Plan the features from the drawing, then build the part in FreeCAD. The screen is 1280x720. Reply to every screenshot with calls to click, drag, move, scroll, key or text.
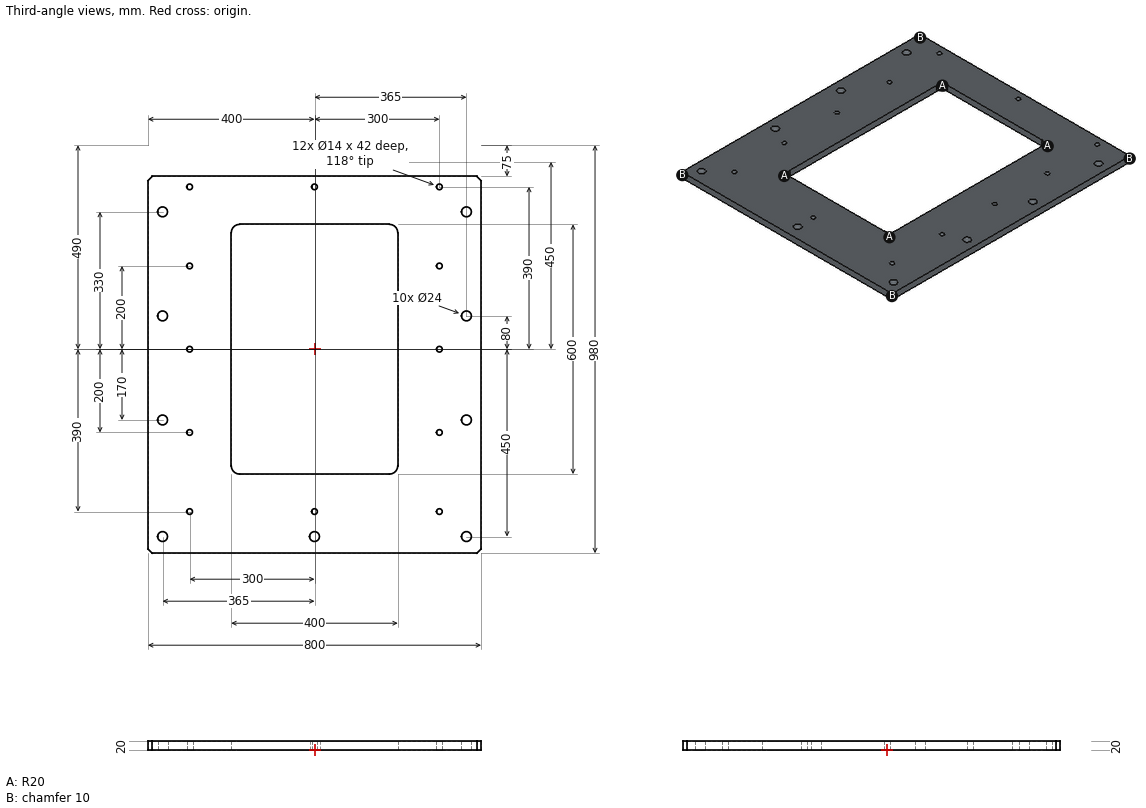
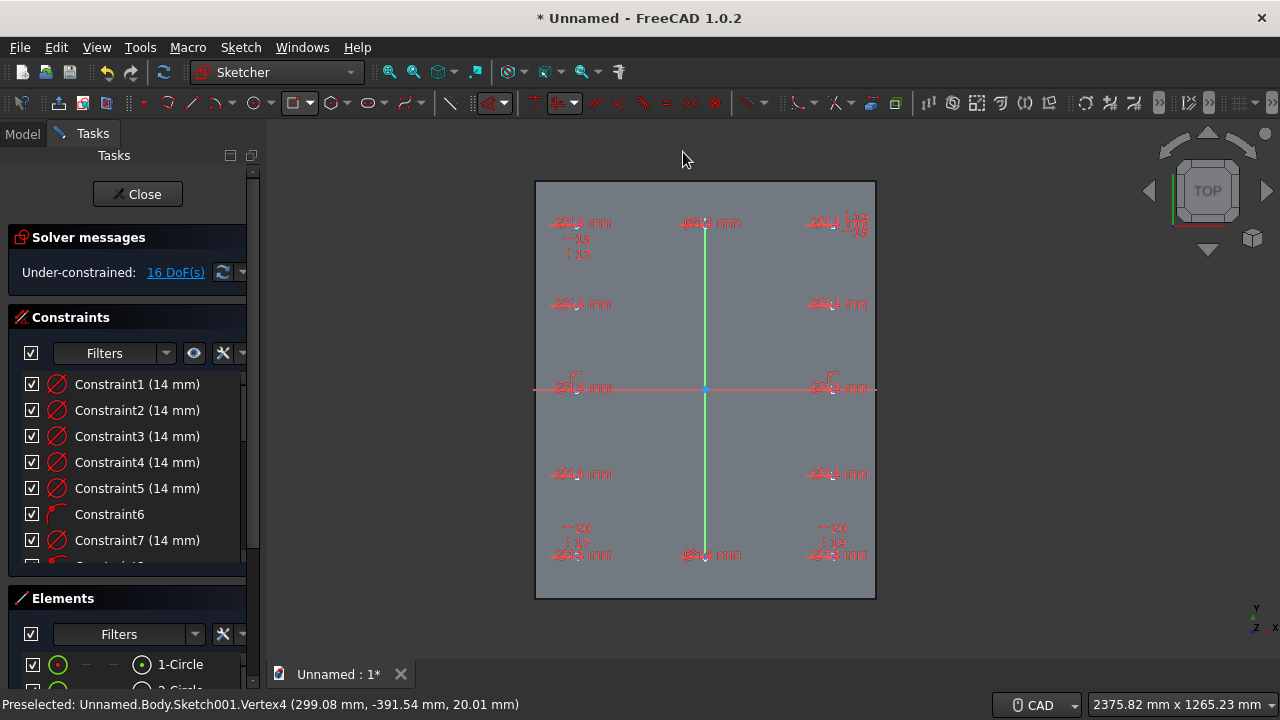
click(577, 557)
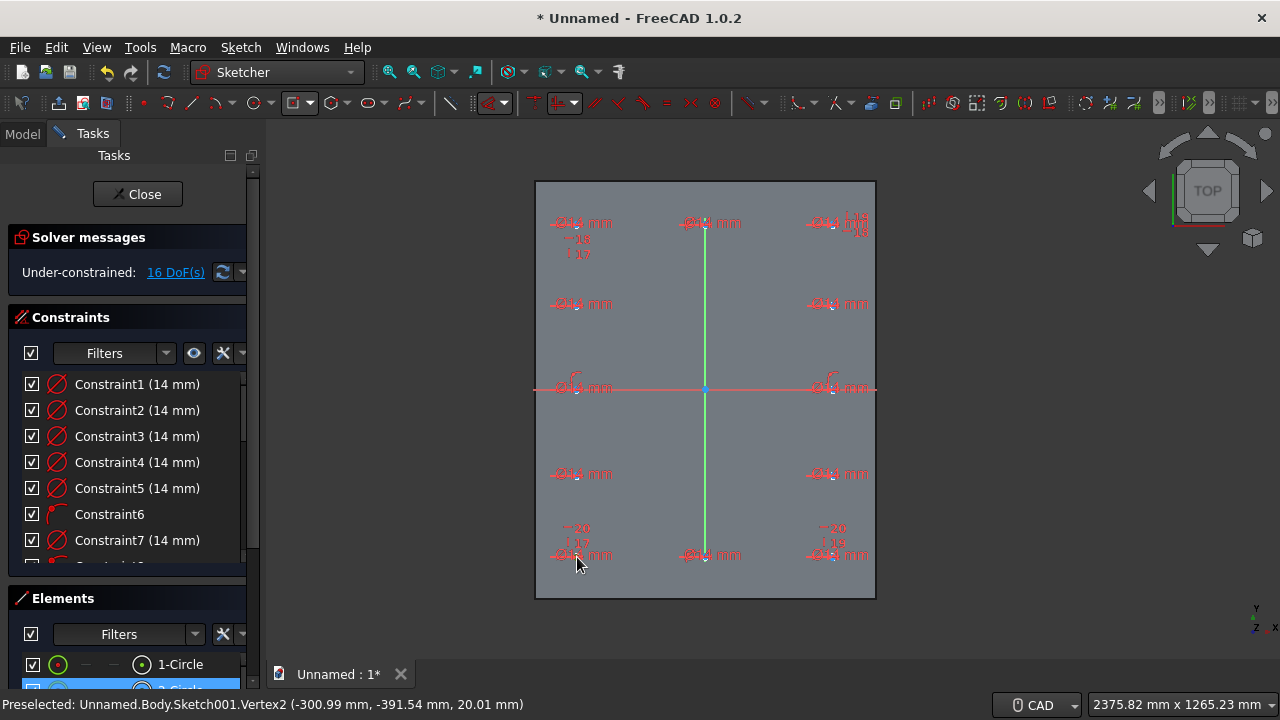
click(577, 390)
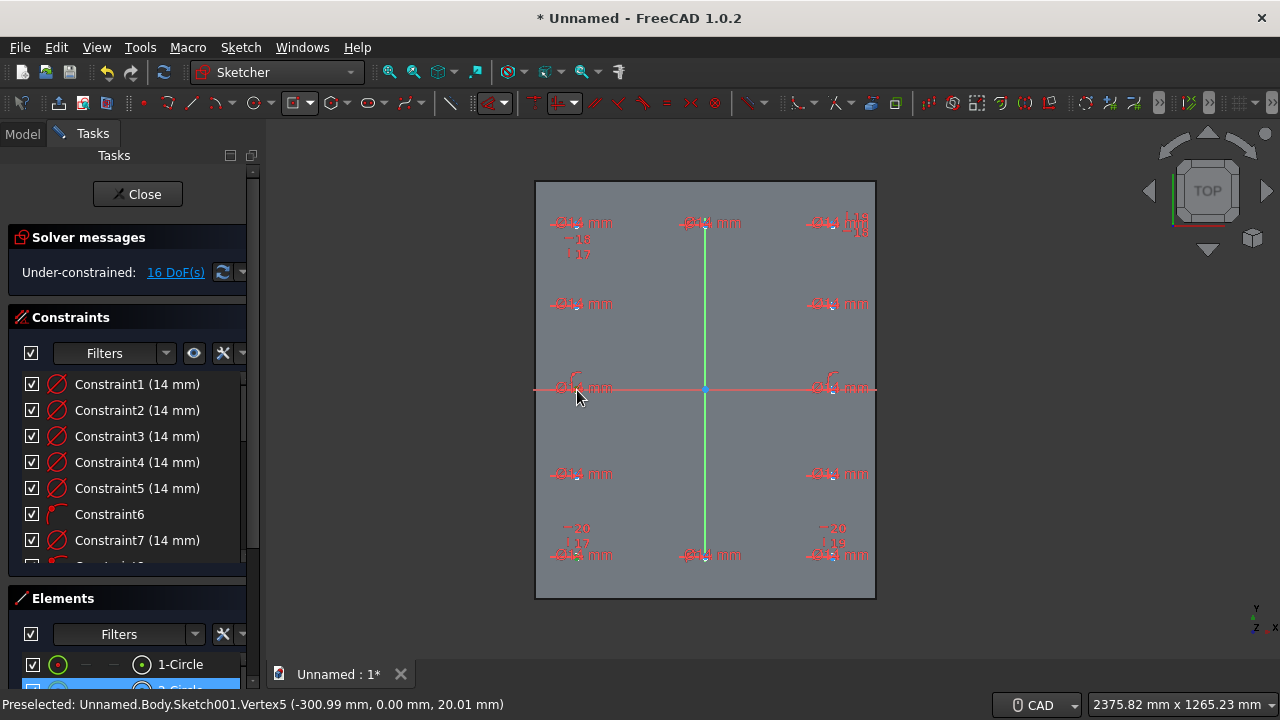
click(576, 104)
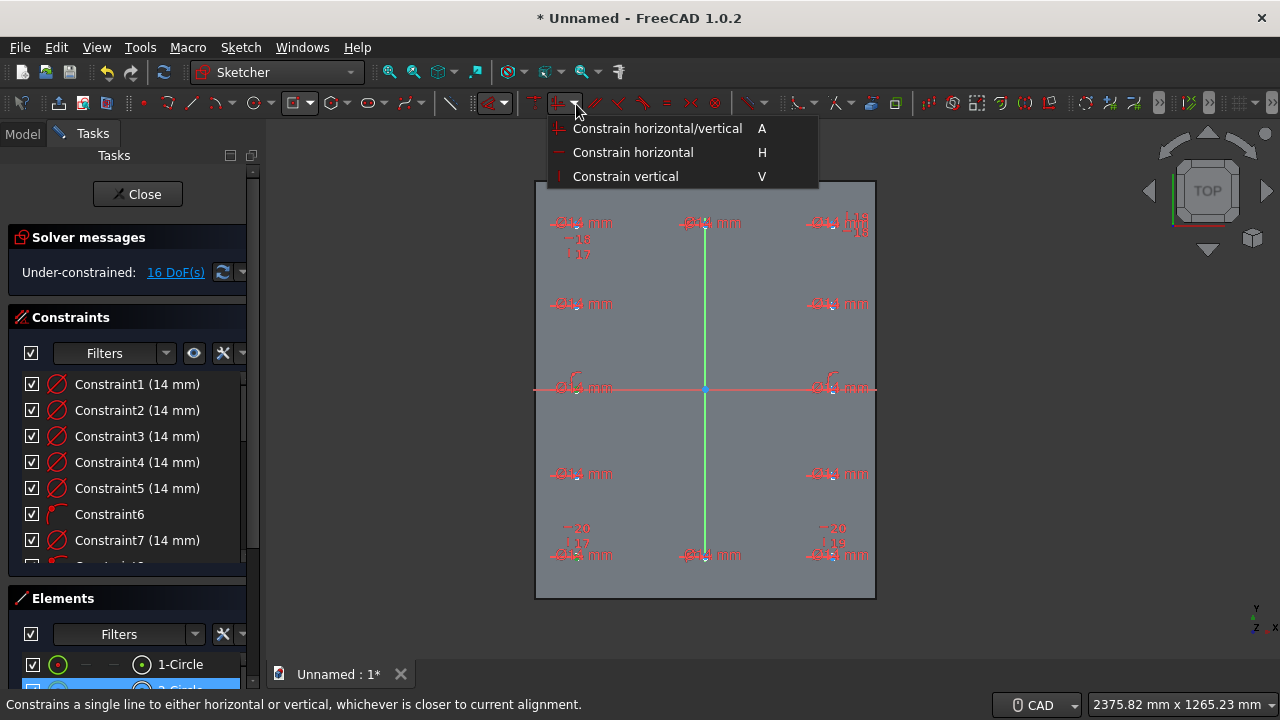
click(683, 176)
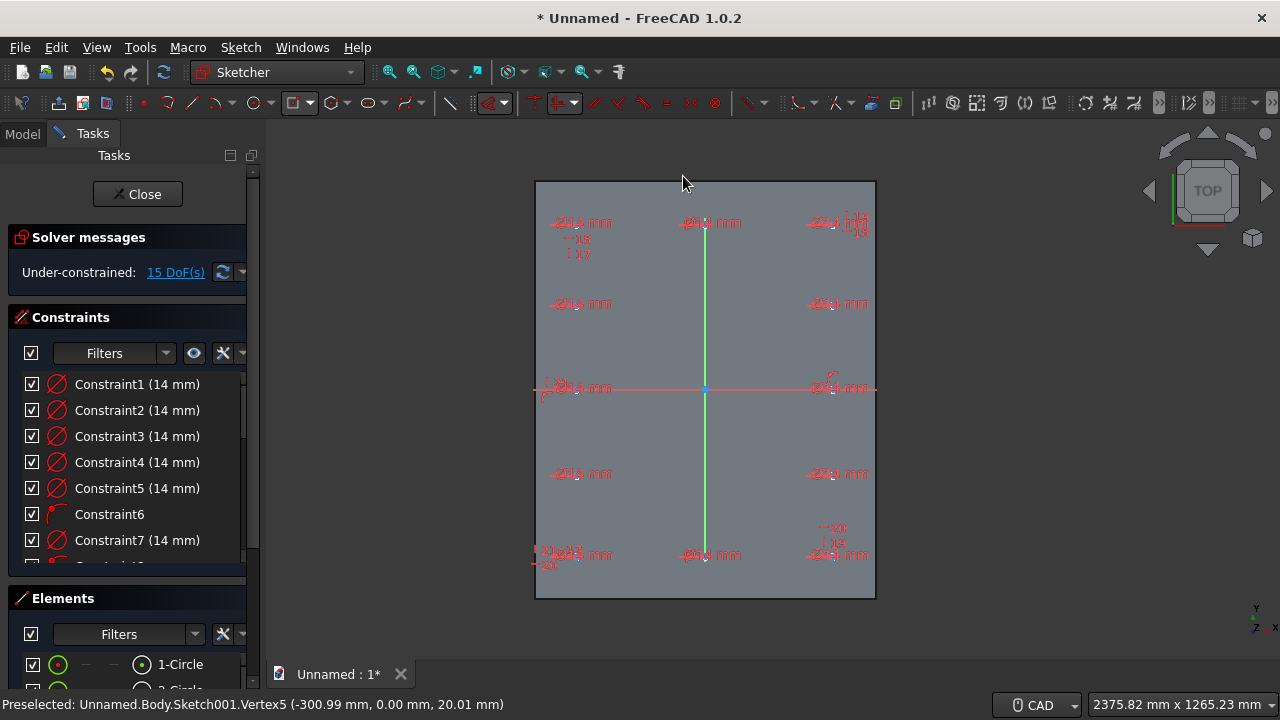
click(577, 557)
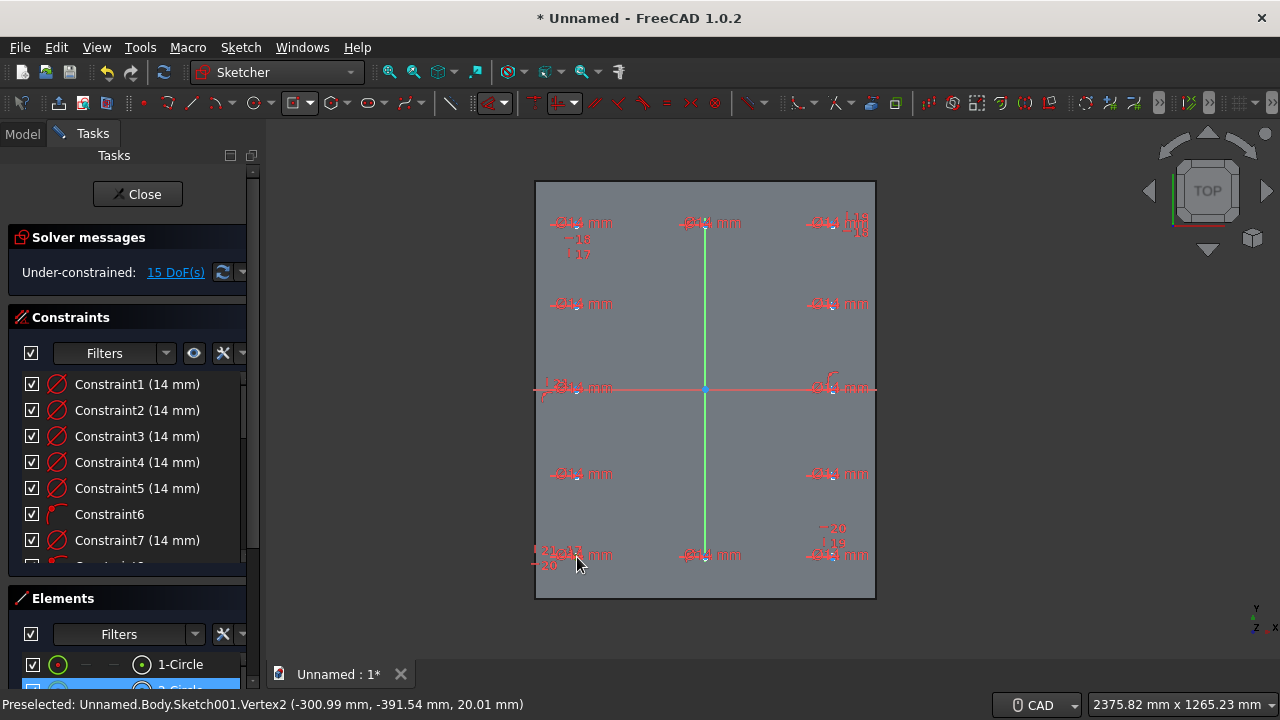
click(705, 557)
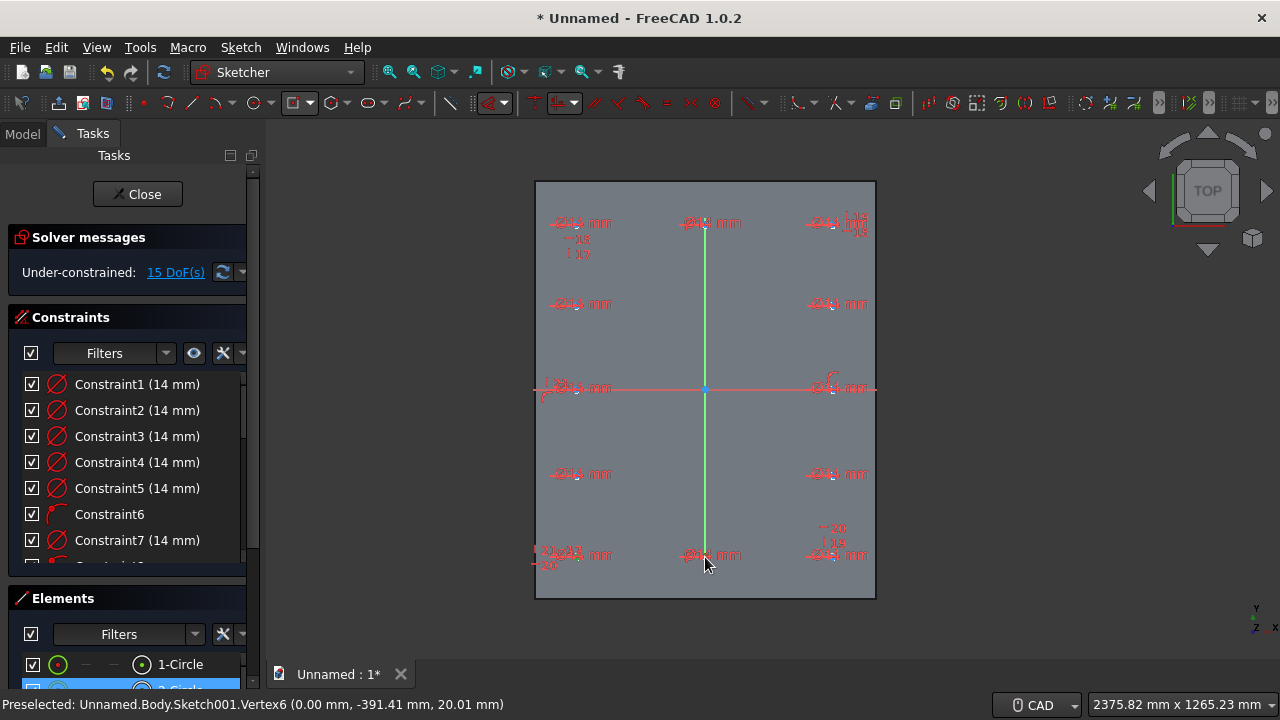
click(576, 104)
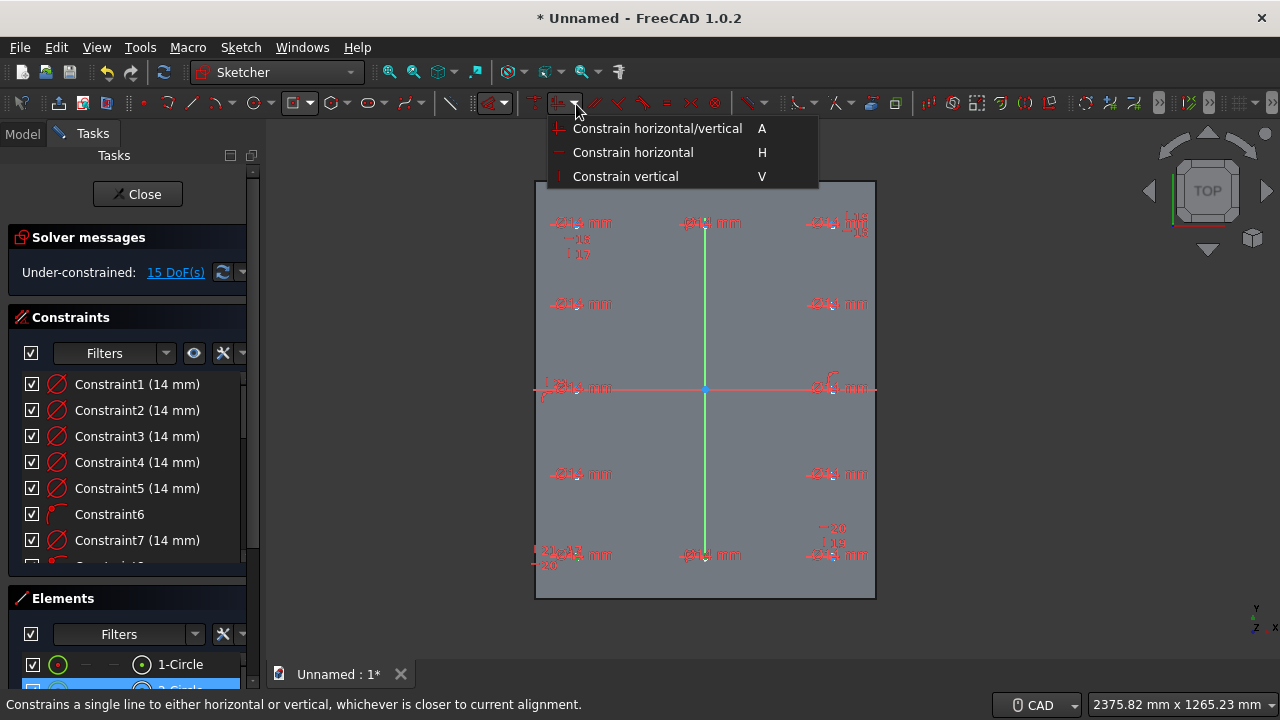
click(683, 152)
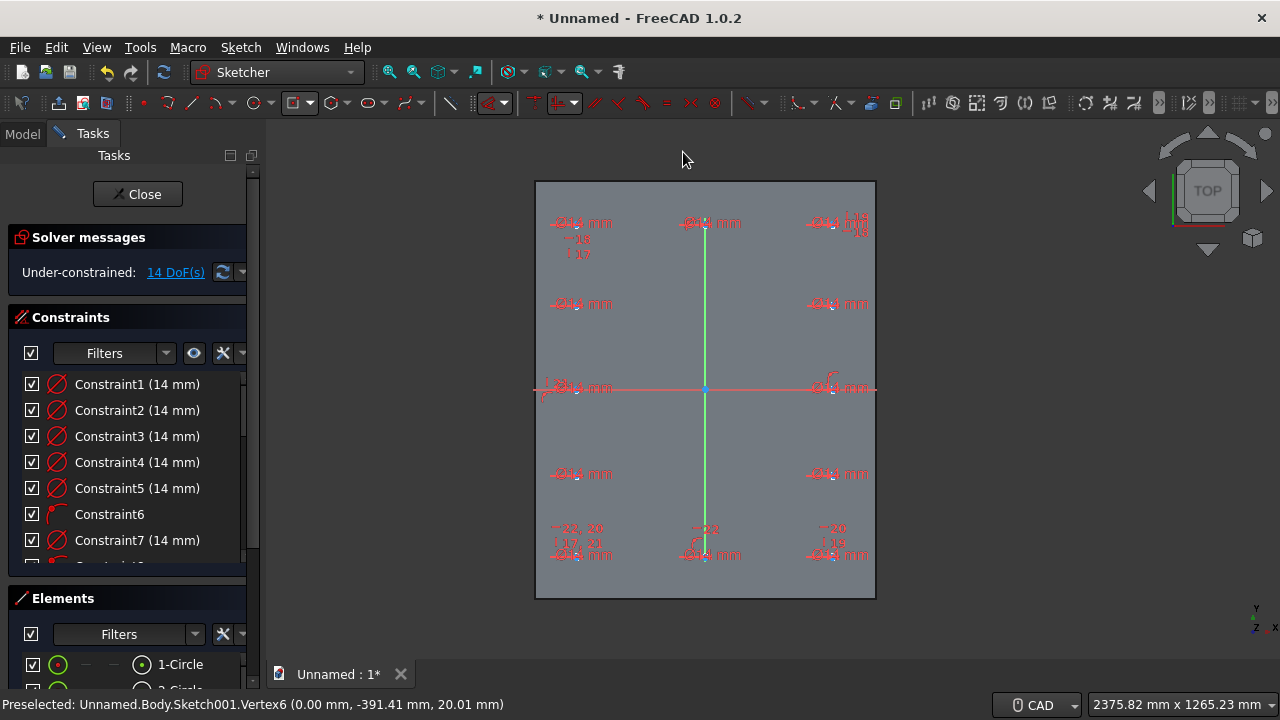
click(833, 225)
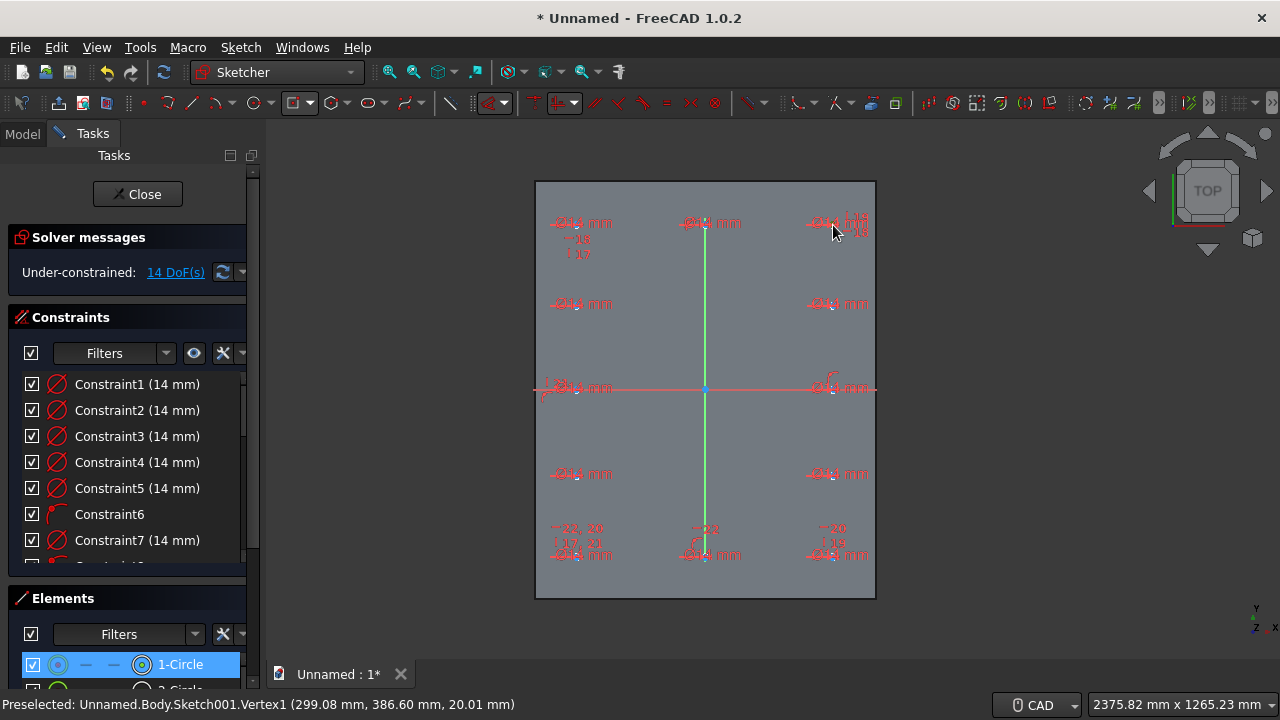
click(833, 390)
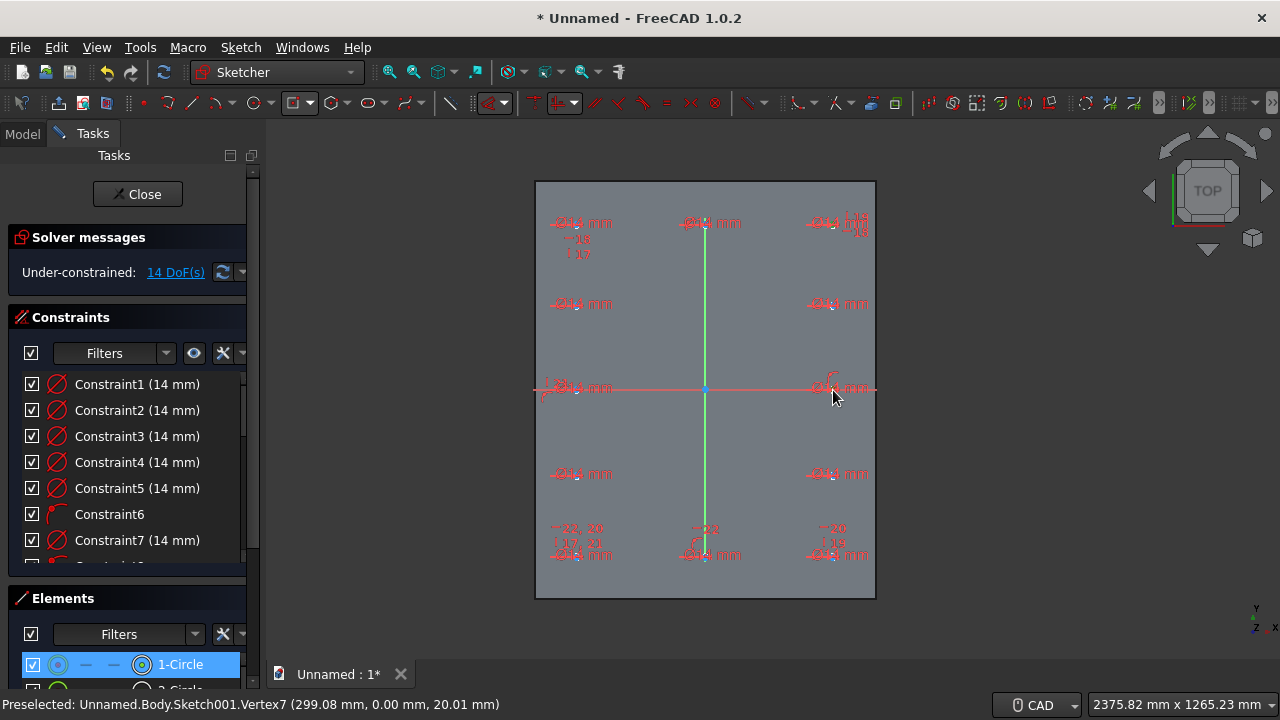
click(576, 104)